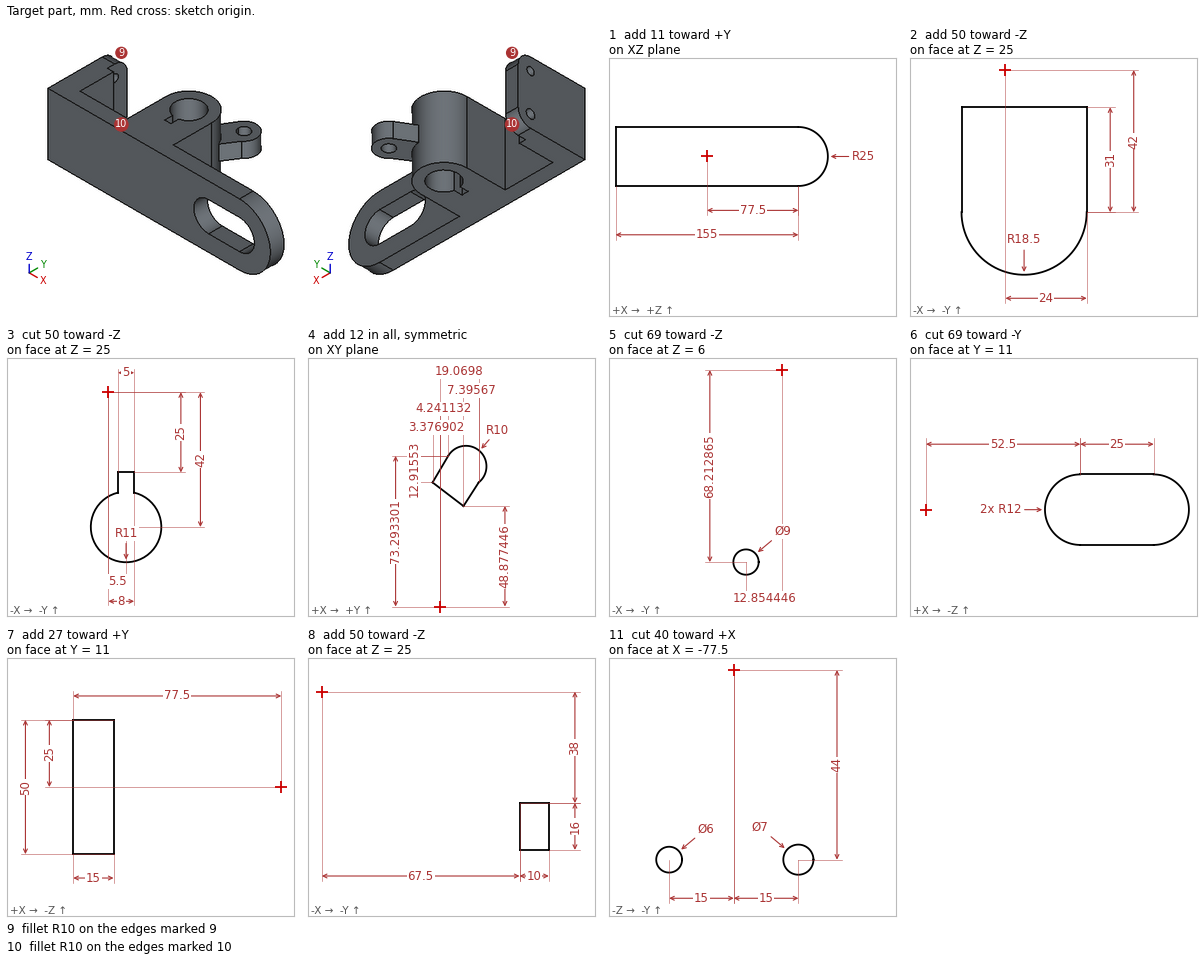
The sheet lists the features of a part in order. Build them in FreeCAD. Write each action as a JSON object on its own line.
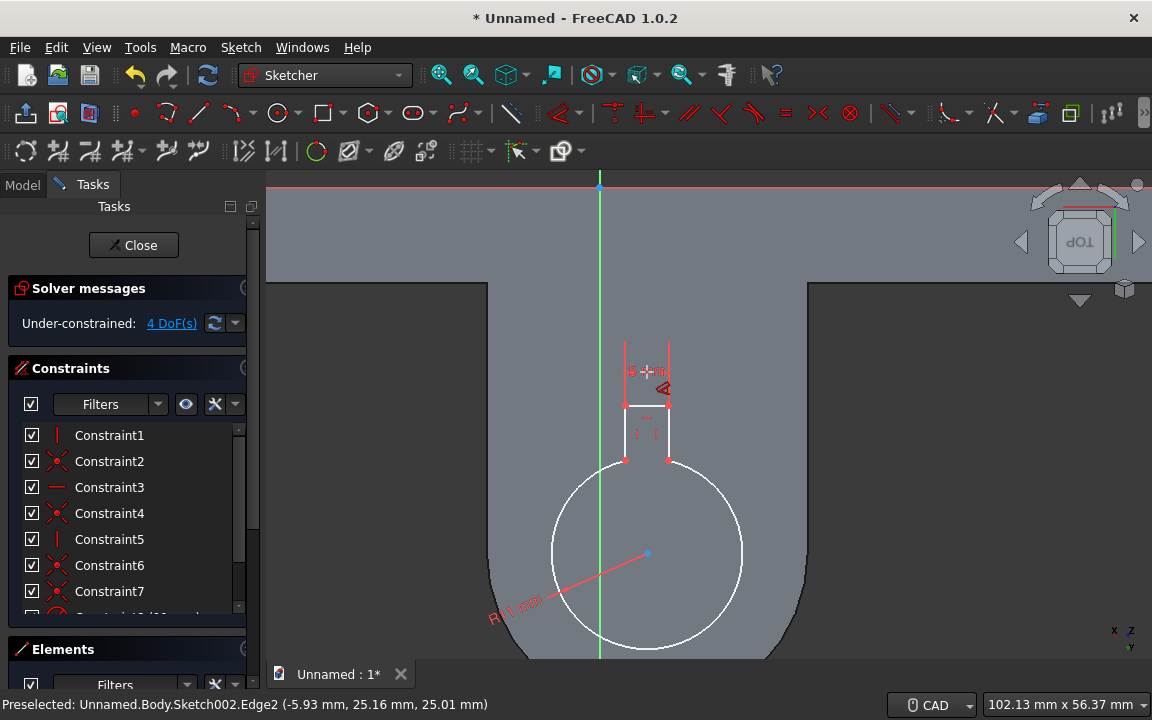
{"action": "left_click", "coordinate": [669, 461]}
{"action": "left_click", "coordinate": [634, 495]}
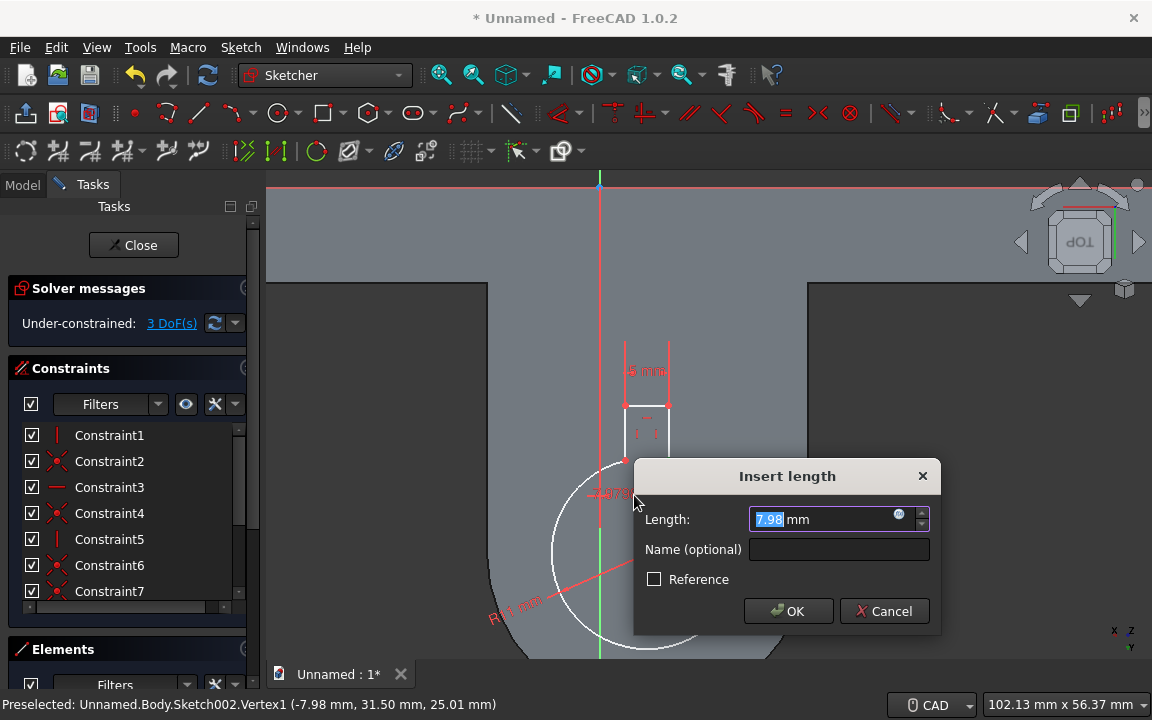
{"action": "type", "text": "8"}
{"action": "key", "text": "Return"}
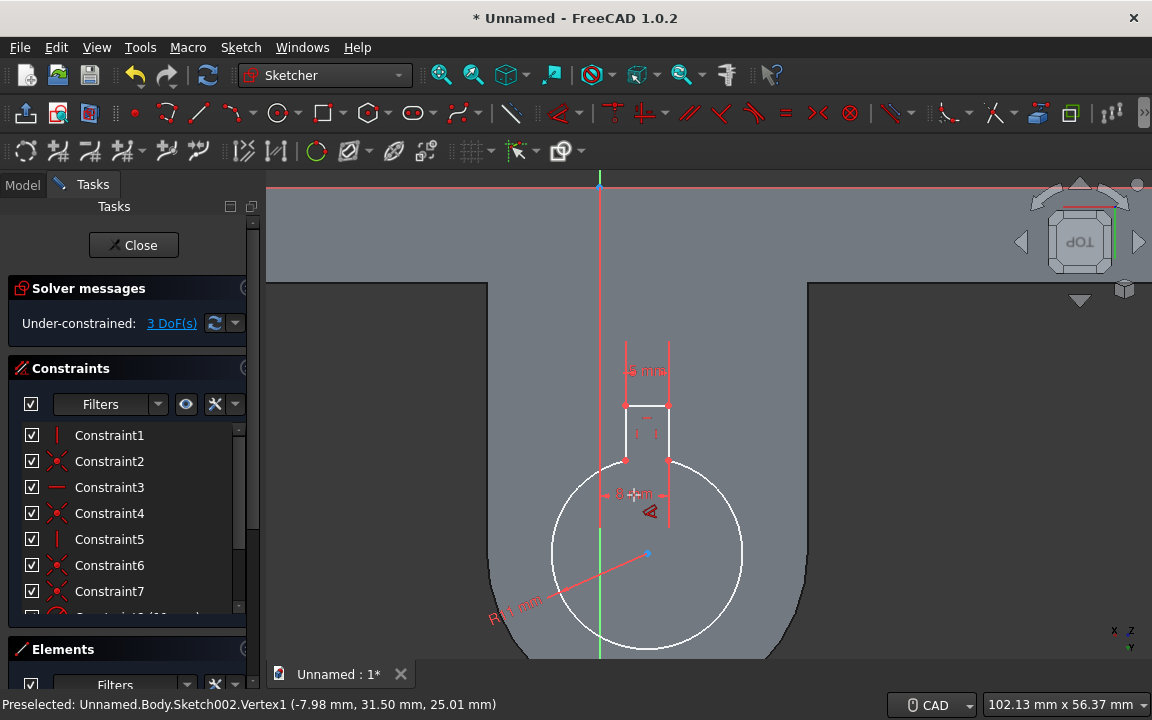
{"action": "left_click", "coordinate": [669, 406]}
{"action": "left_click", "coordinate": [703, 302]}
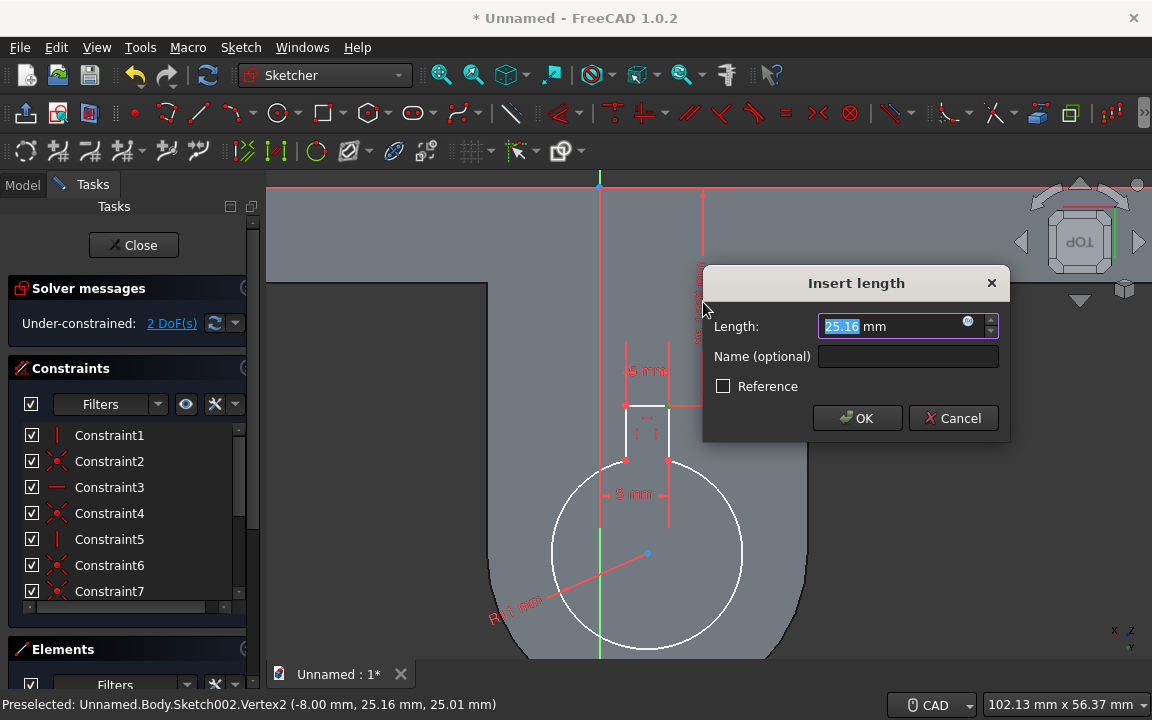
{"action": "type", "text": "25"}
{"action": "key", "text": "Return"}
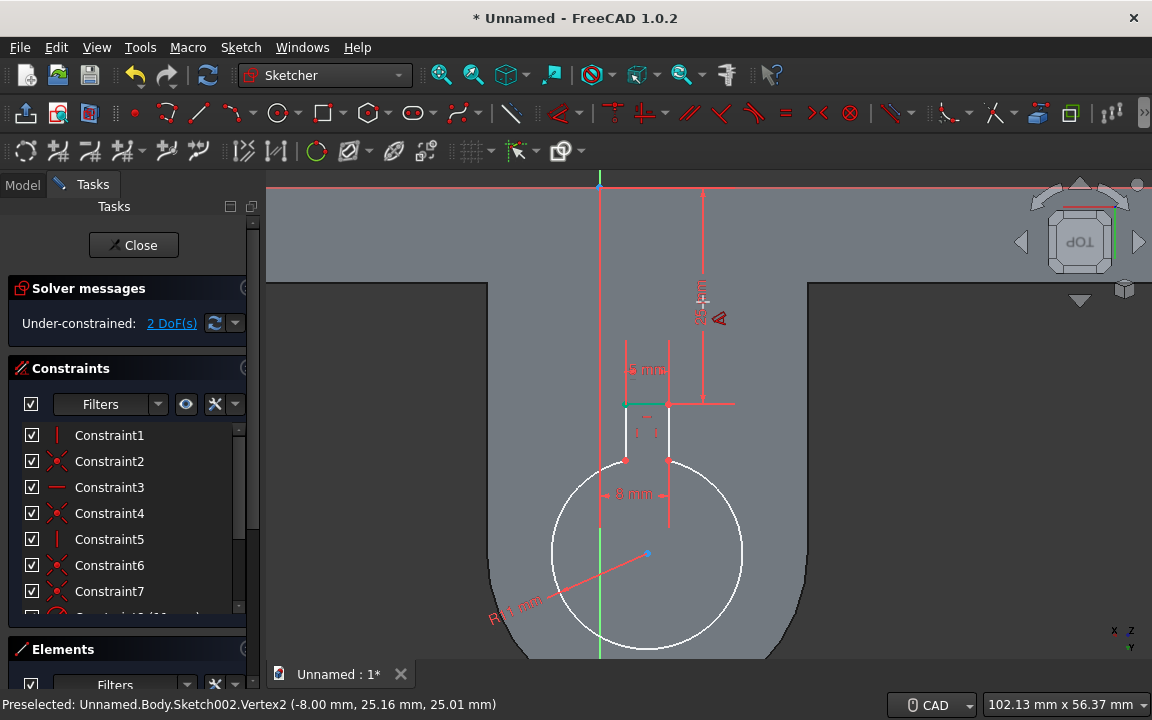
{"action": "left_click", "coordinate": [647, 554]}
{"action": "left_click", "coordinate": [566, 376]}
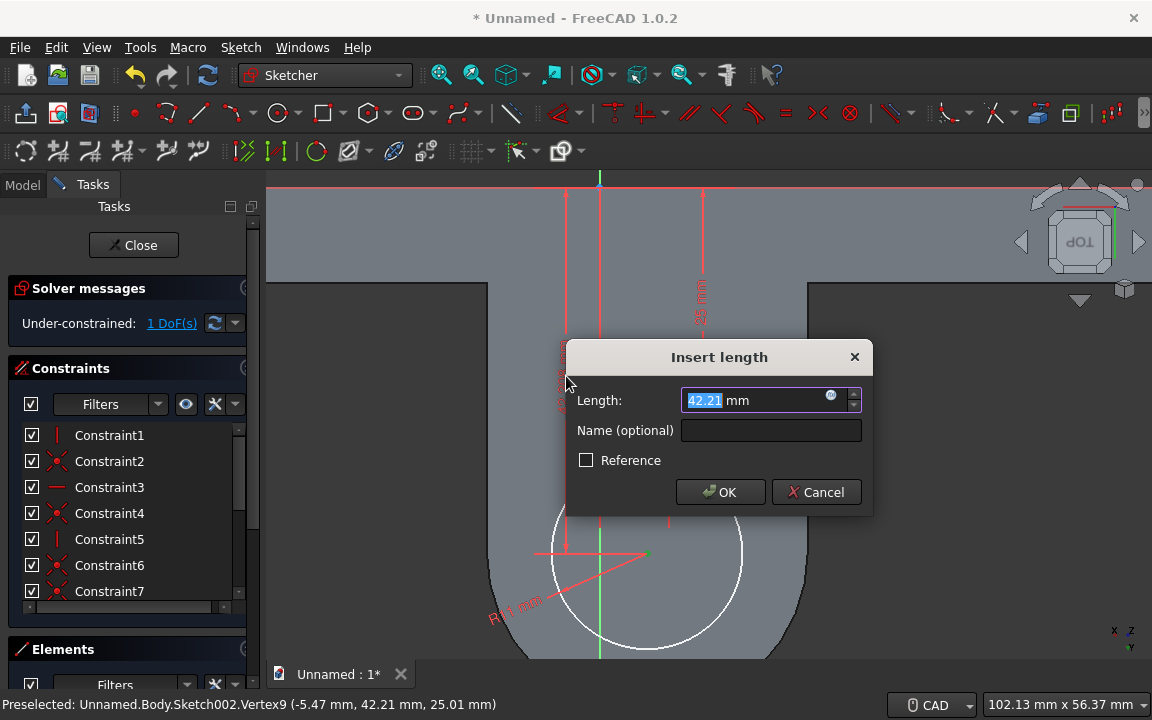
{"action": "type", "text": "42"}
{"action": "key", "text": "Return"}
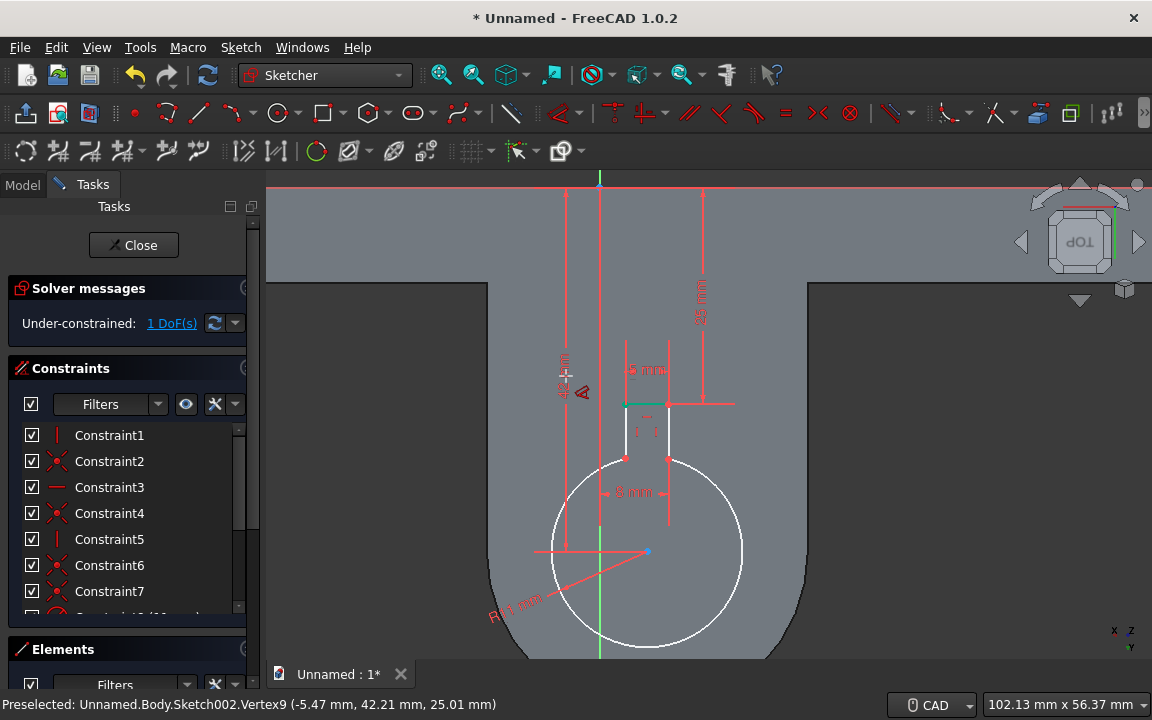
{"action": "left_click", "coordinate": [647, 552]}
{"action": "left_click", "coordinate": [623, 586]}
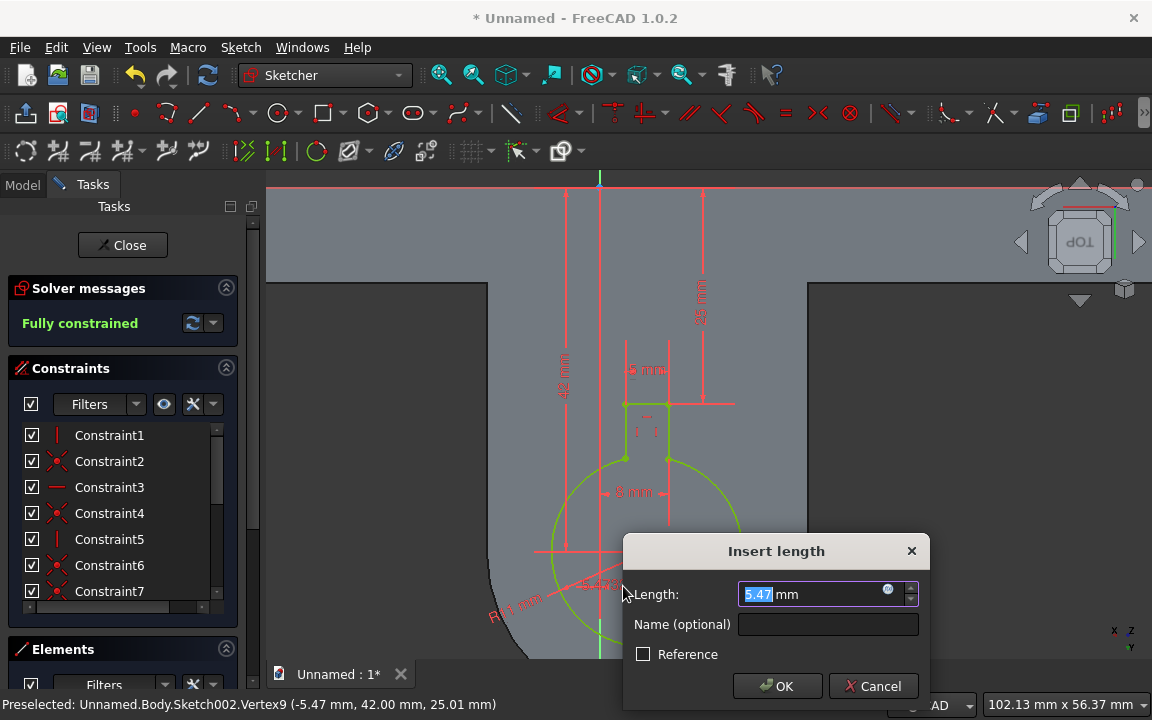
{"action": "type", "text": "5.5"}
{"action": "key", "text": "Return"}
{"action": "key", "text": "Escape"}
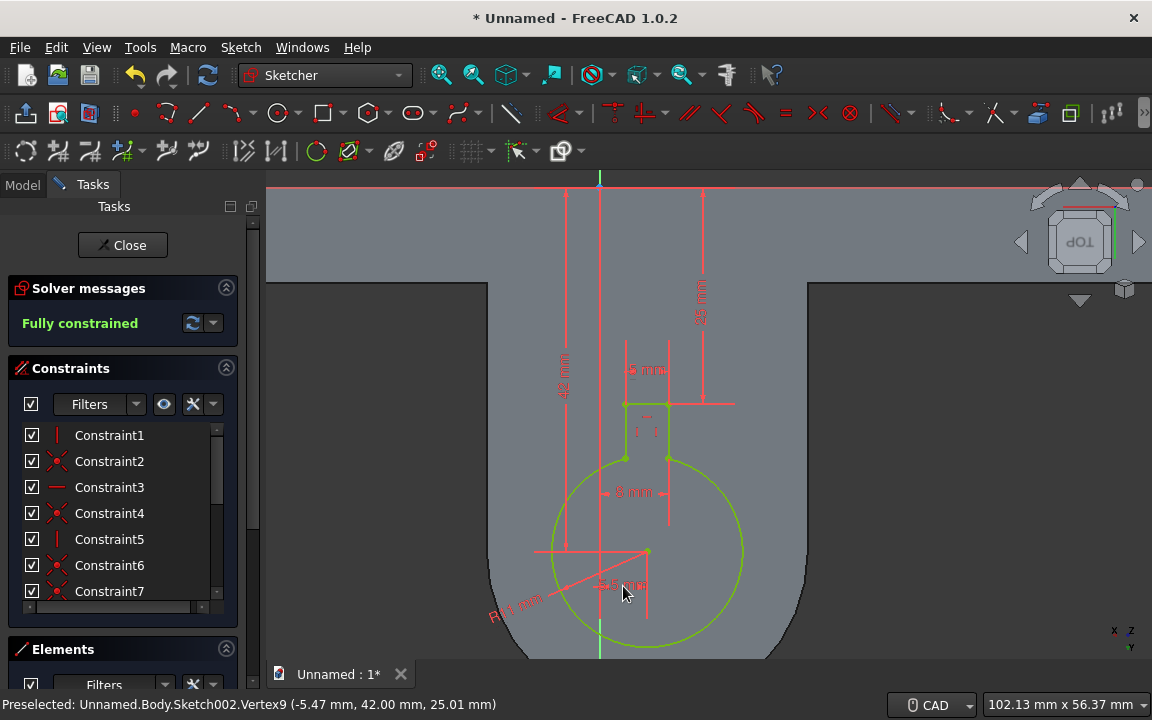
{"action": "left_click", "coordinate": [123, 245]}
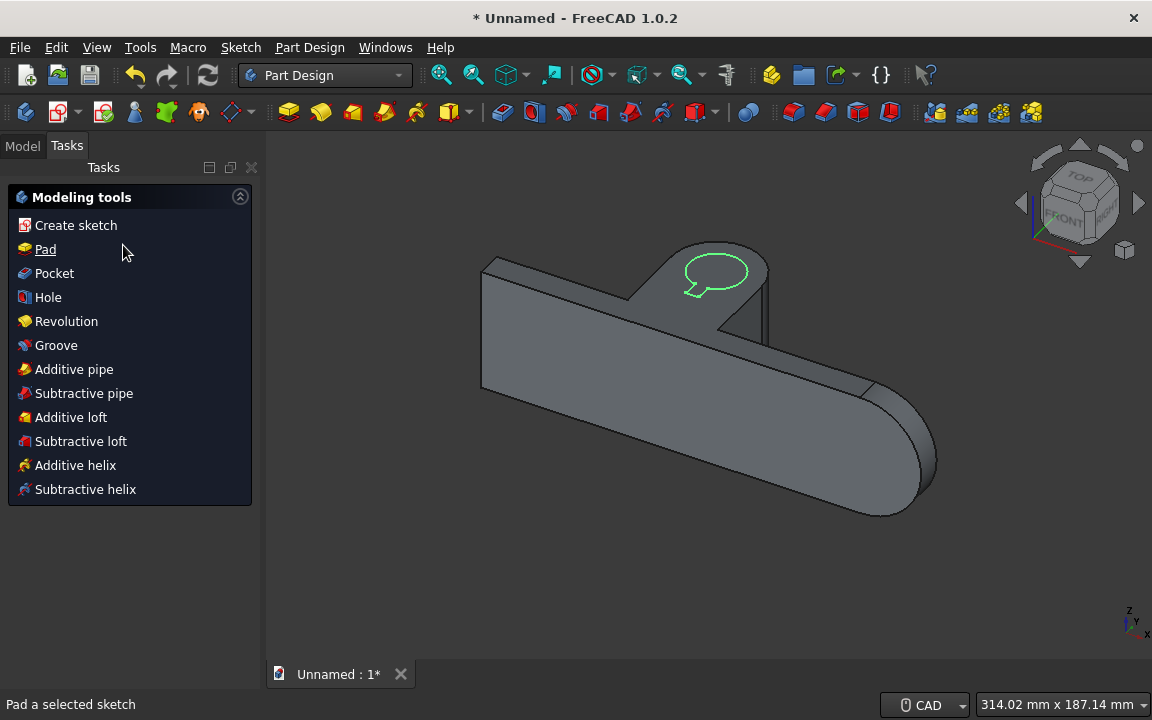
{"action": "left_click", "coordinate": [504, 112]}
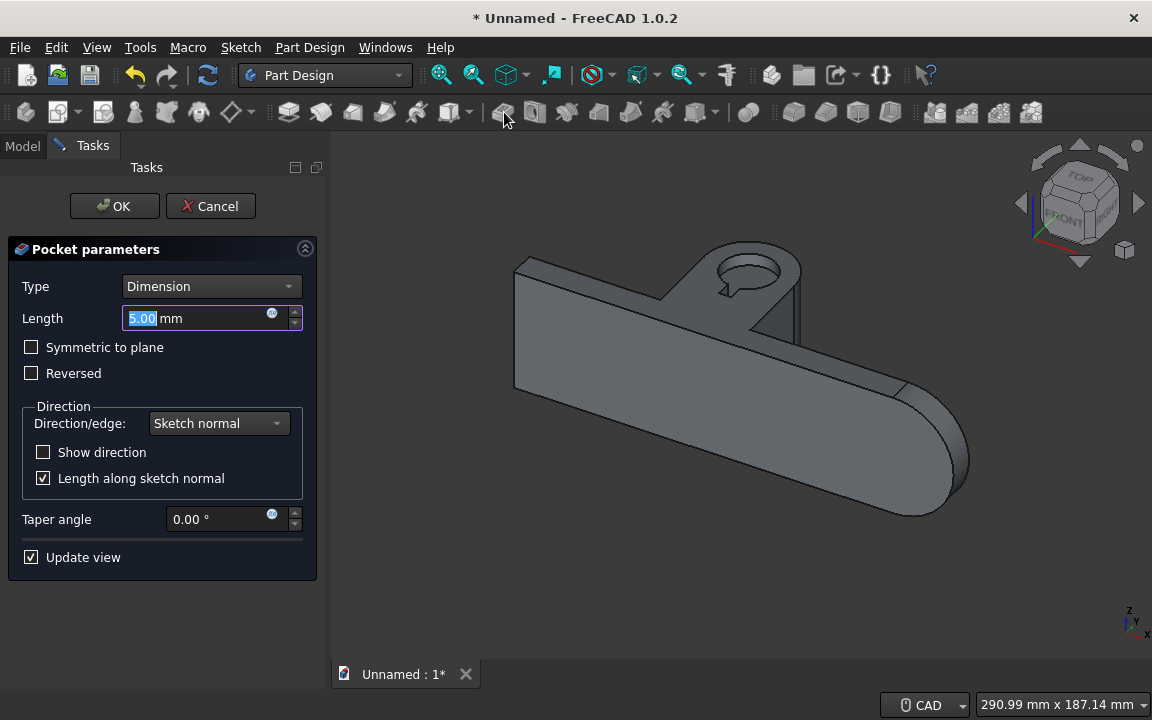
{"action": "type", "text": "50"}
{"action": "key", "text": "Tab"}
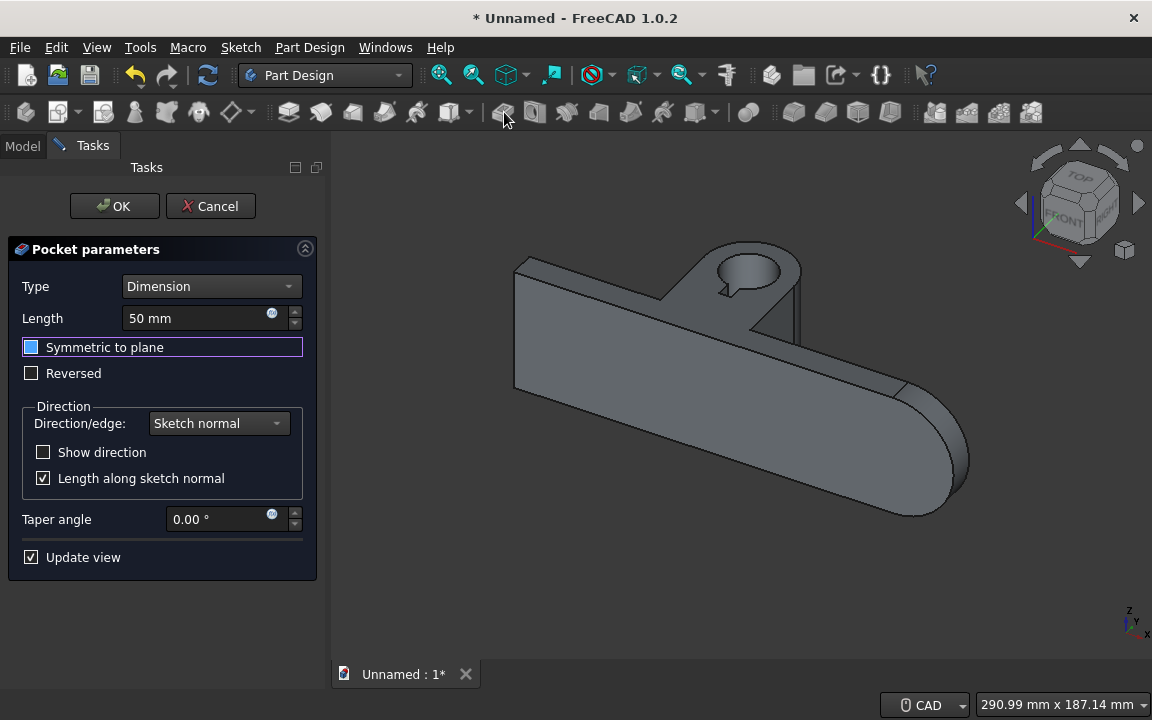
{"action": "left_click", "coordinate": [115, 206]}